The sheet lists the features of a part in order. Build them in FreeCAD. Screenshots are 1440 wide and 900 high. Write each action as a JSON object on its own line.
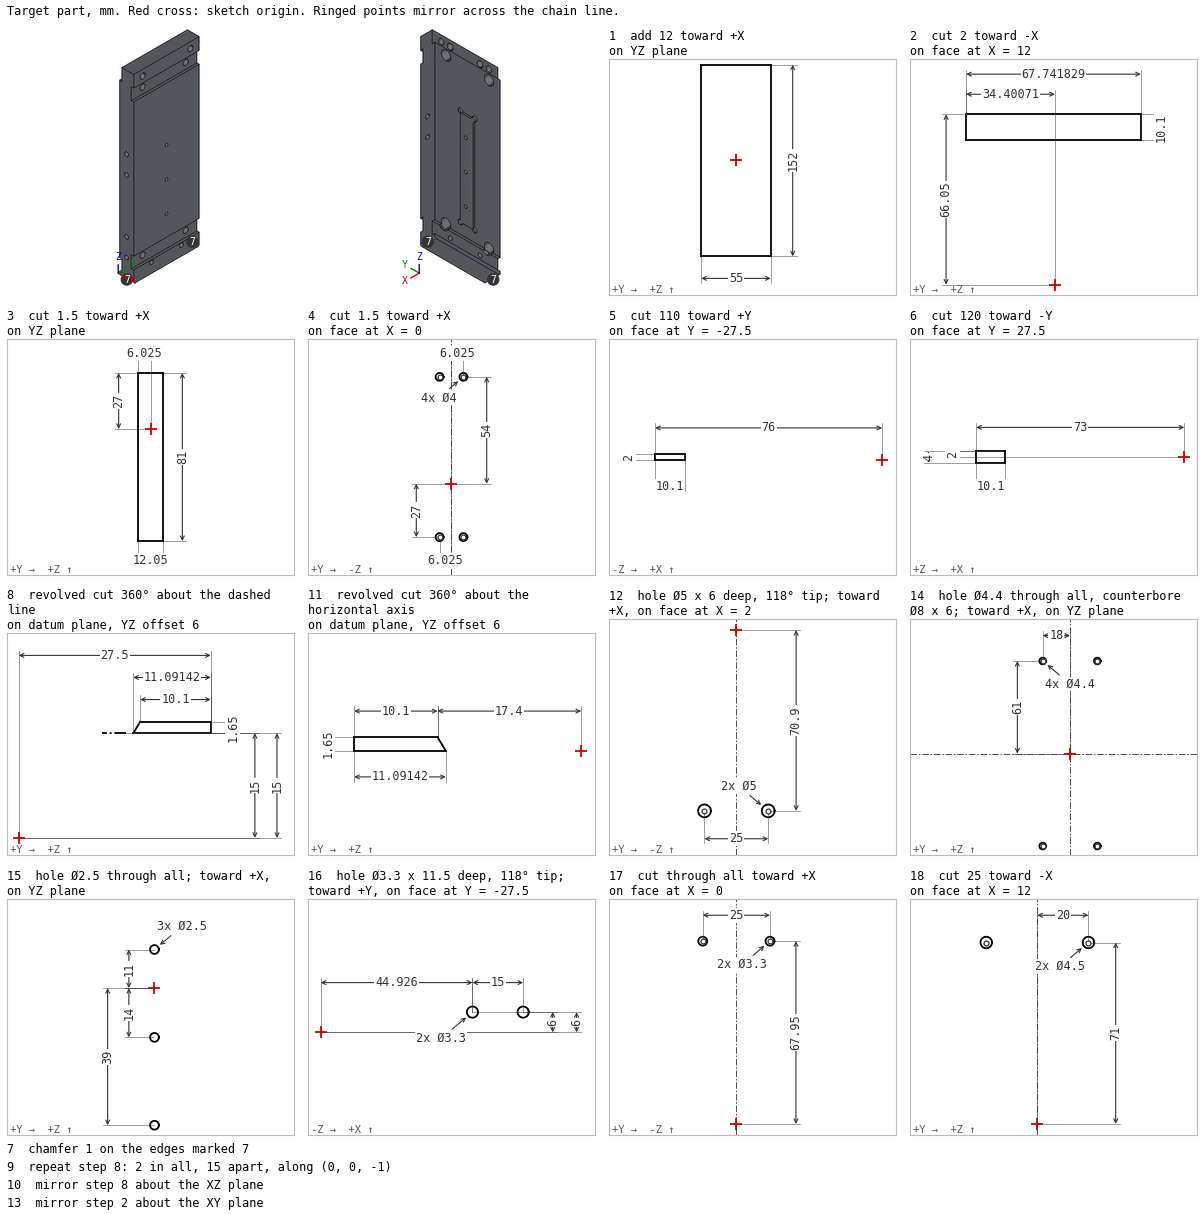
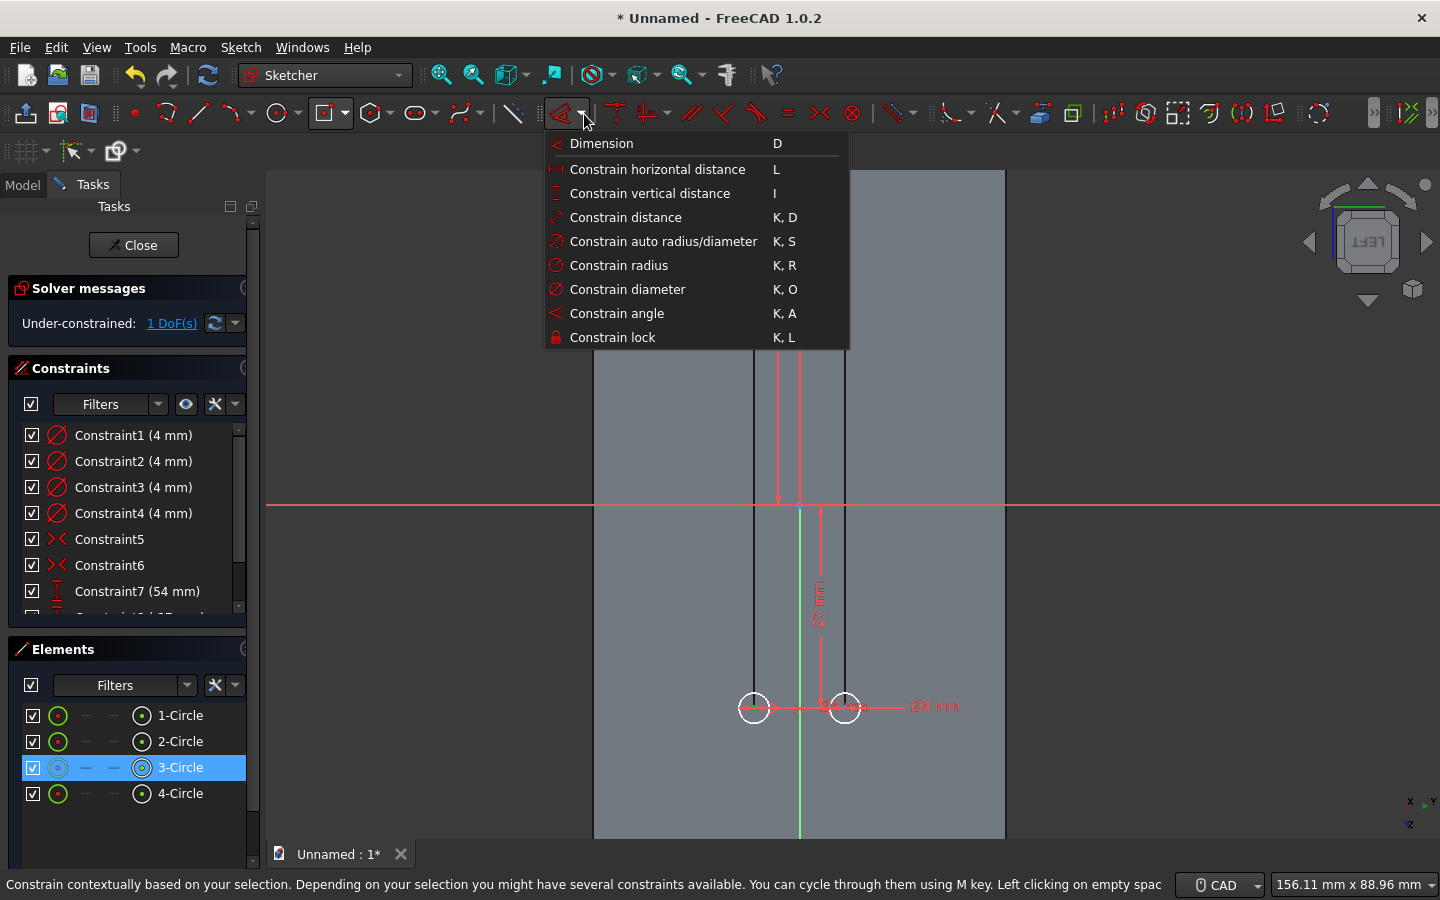
{"action": "left_click", "coordinate": [697, 169]}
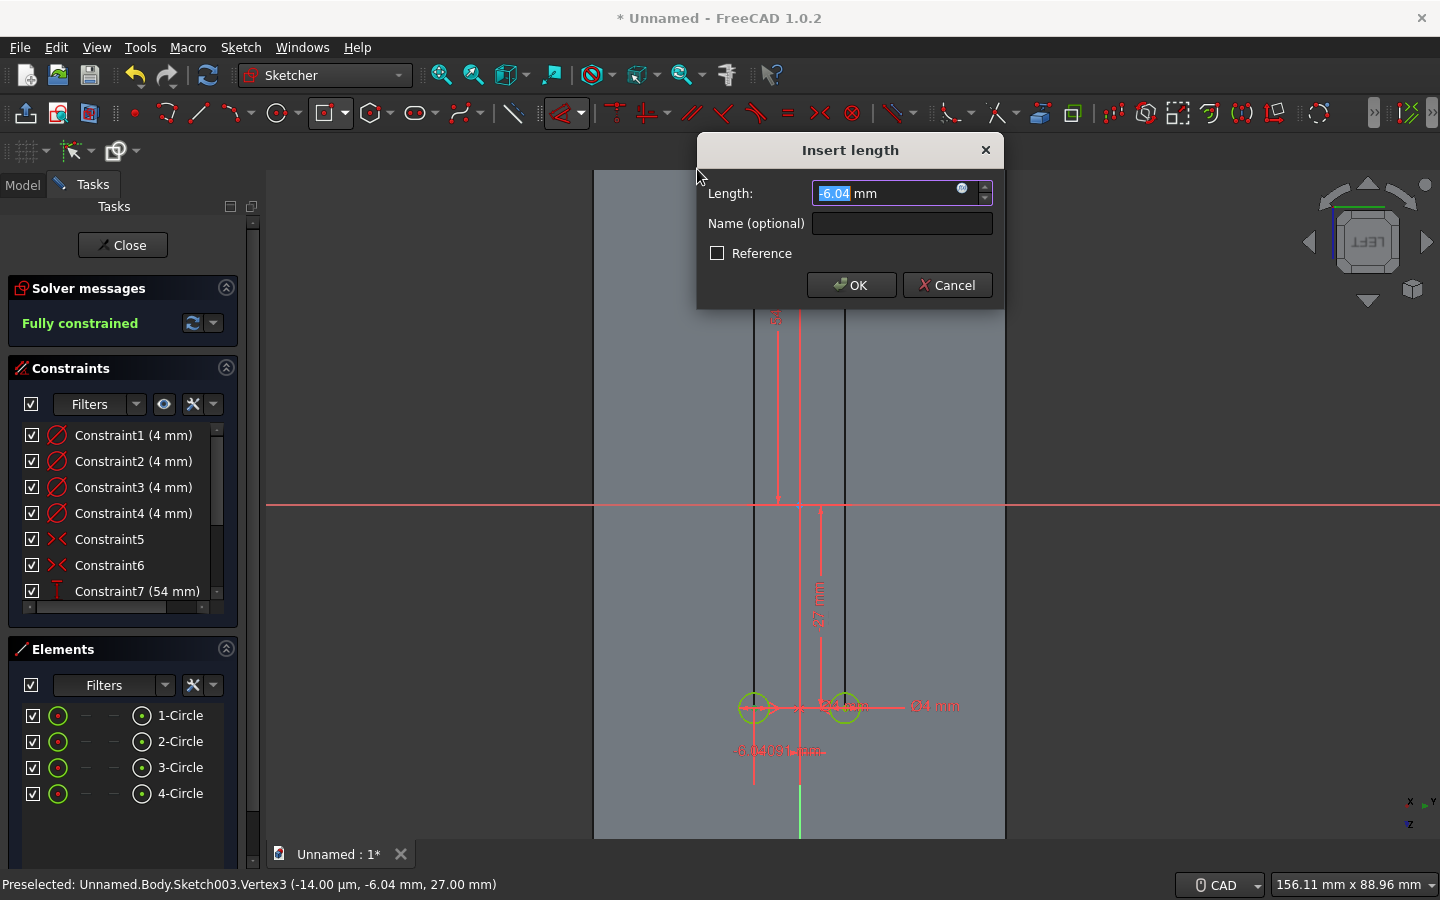
{"action": "type", "text": "-6.025"}
{"action": "key", "text": "Return"}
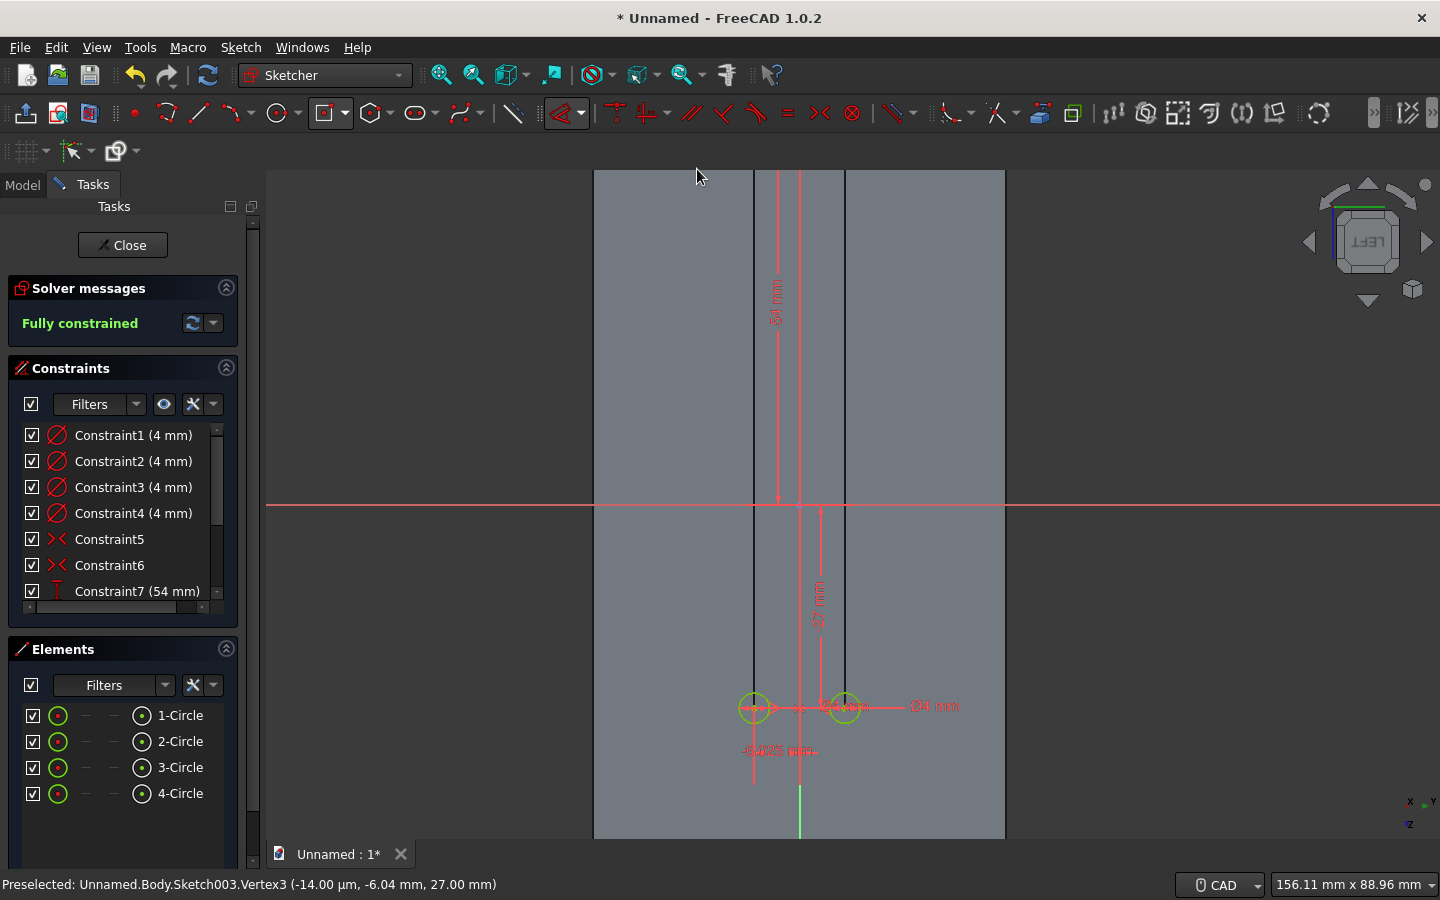
{"action": "left_click", "coordinate": [123, 245]}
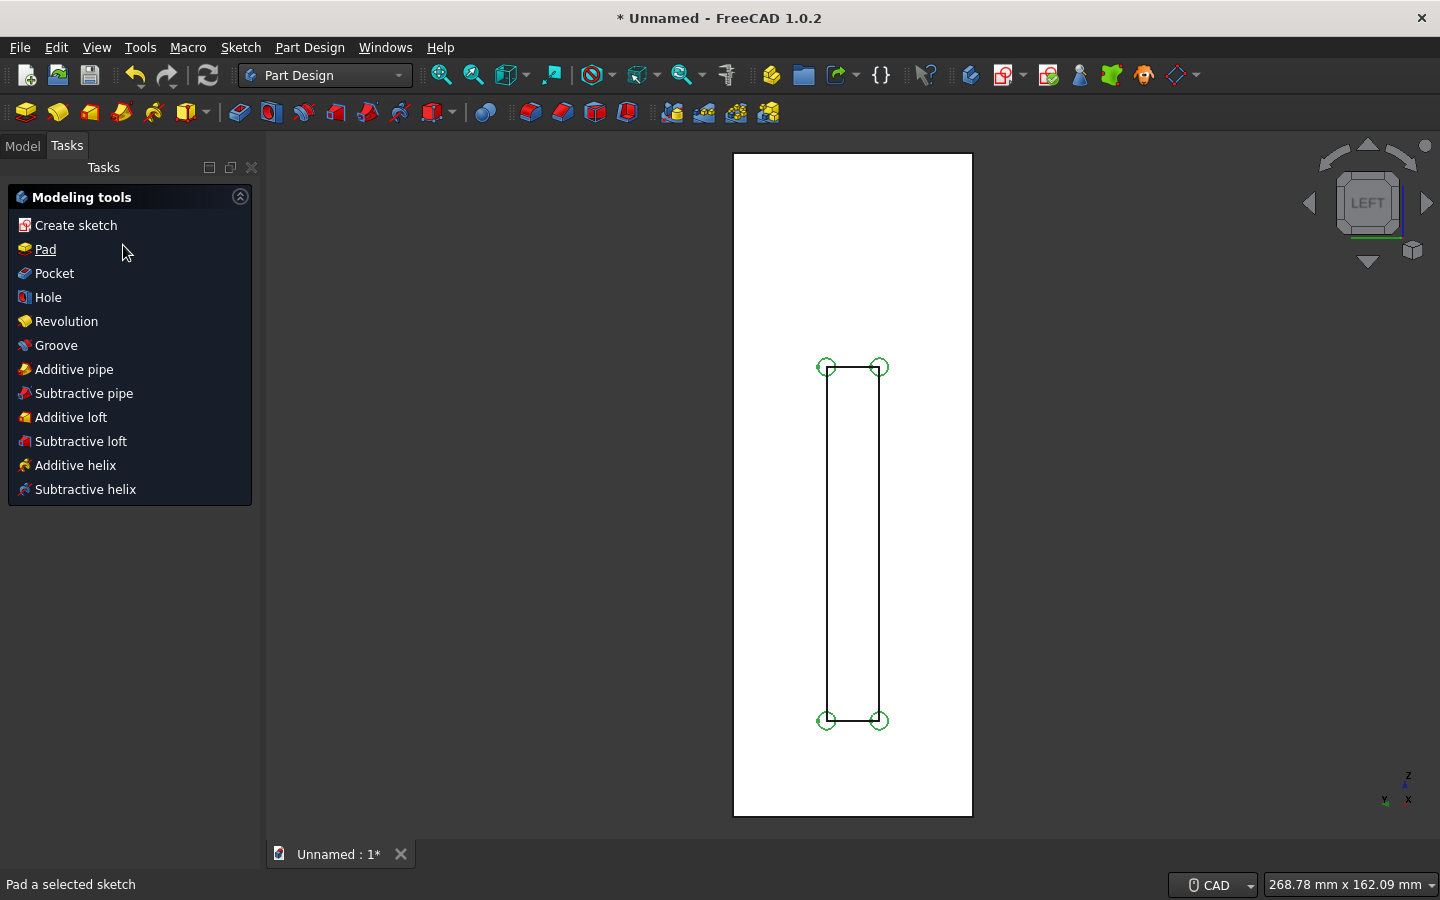
{"action": "left_click", "coordinate": [240, 112]}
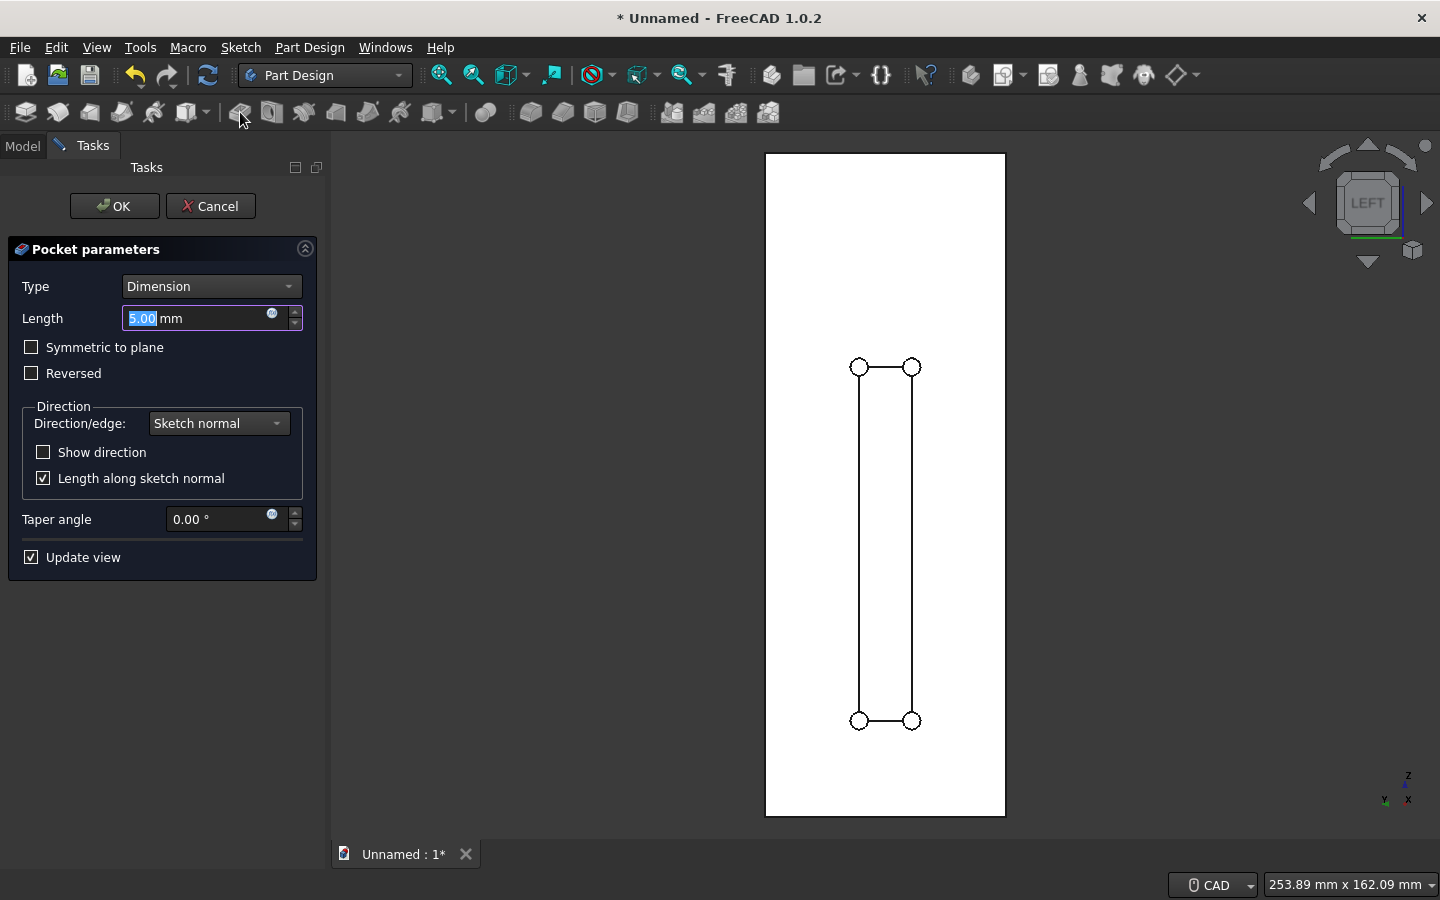
{"action": "type", "text": "1.5"}
{"action": "key", "text": "Tab"}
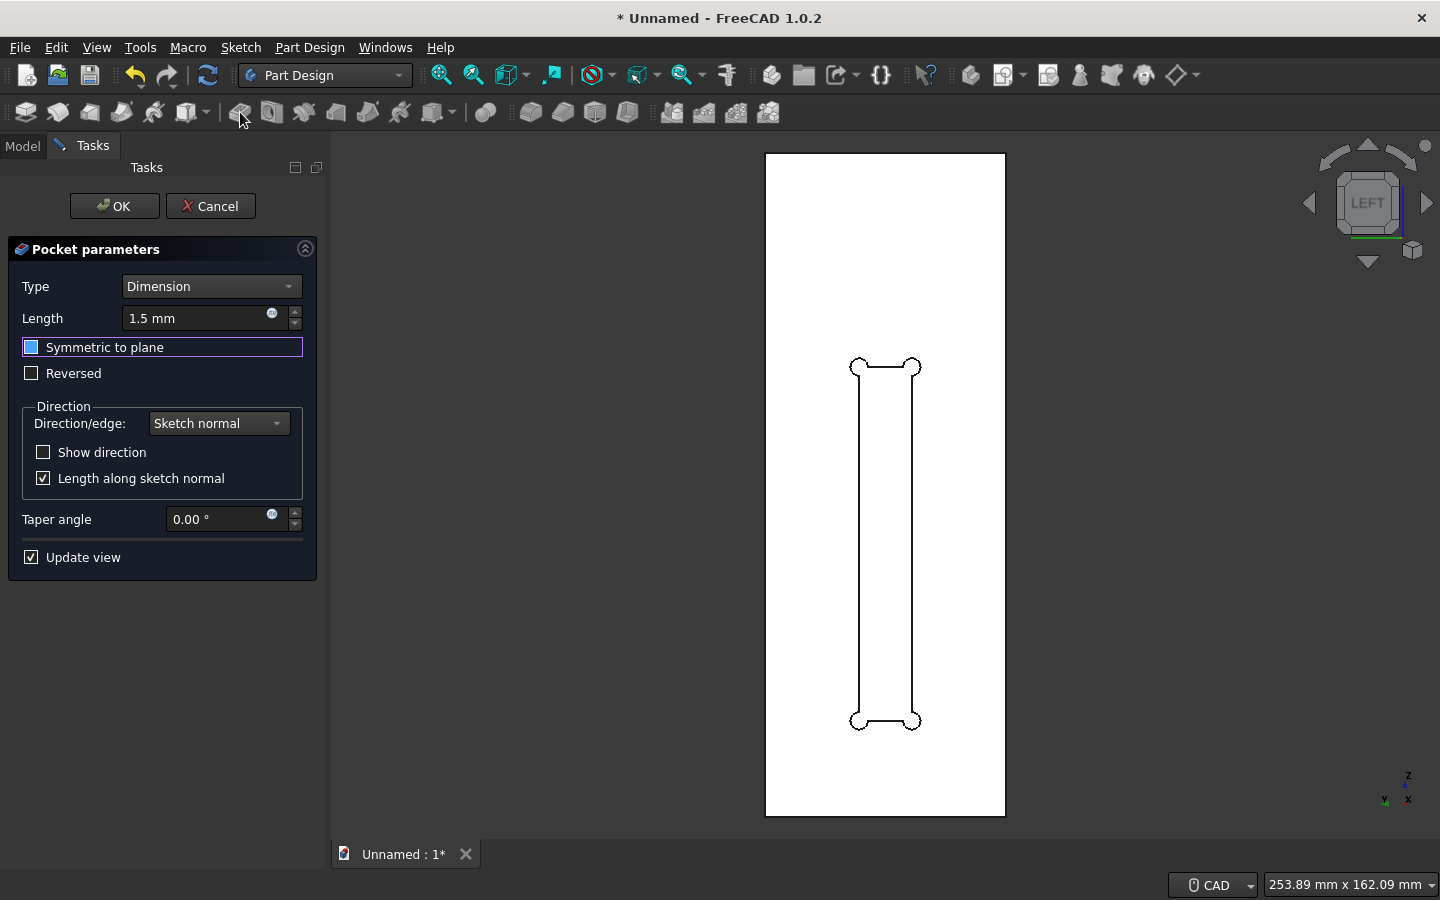
{"action": "left_click", "coordinate": [115, 206]}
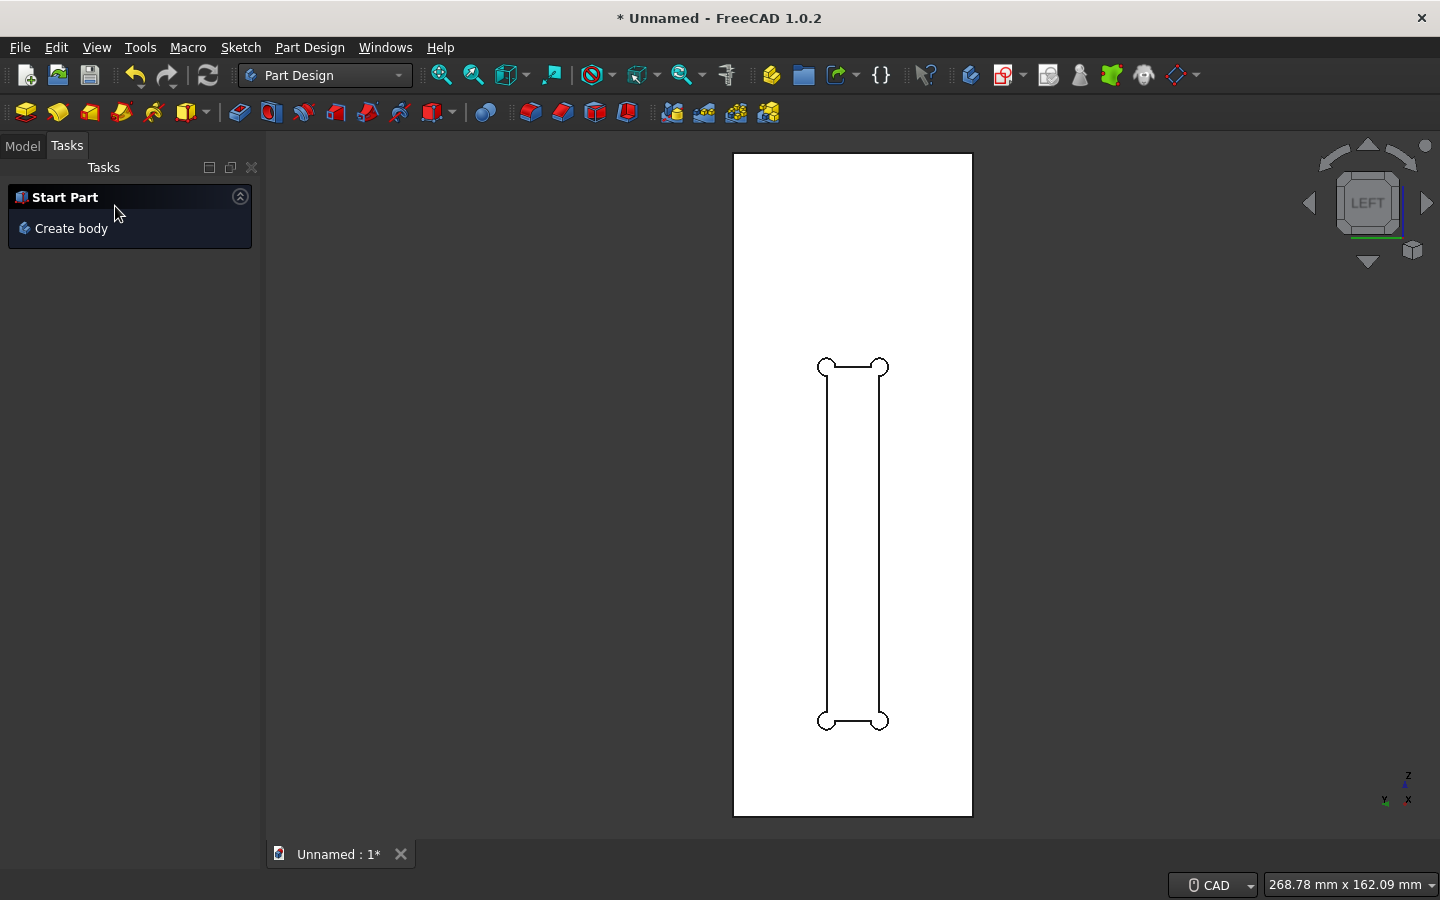
{"action": "key", "text": "0"}